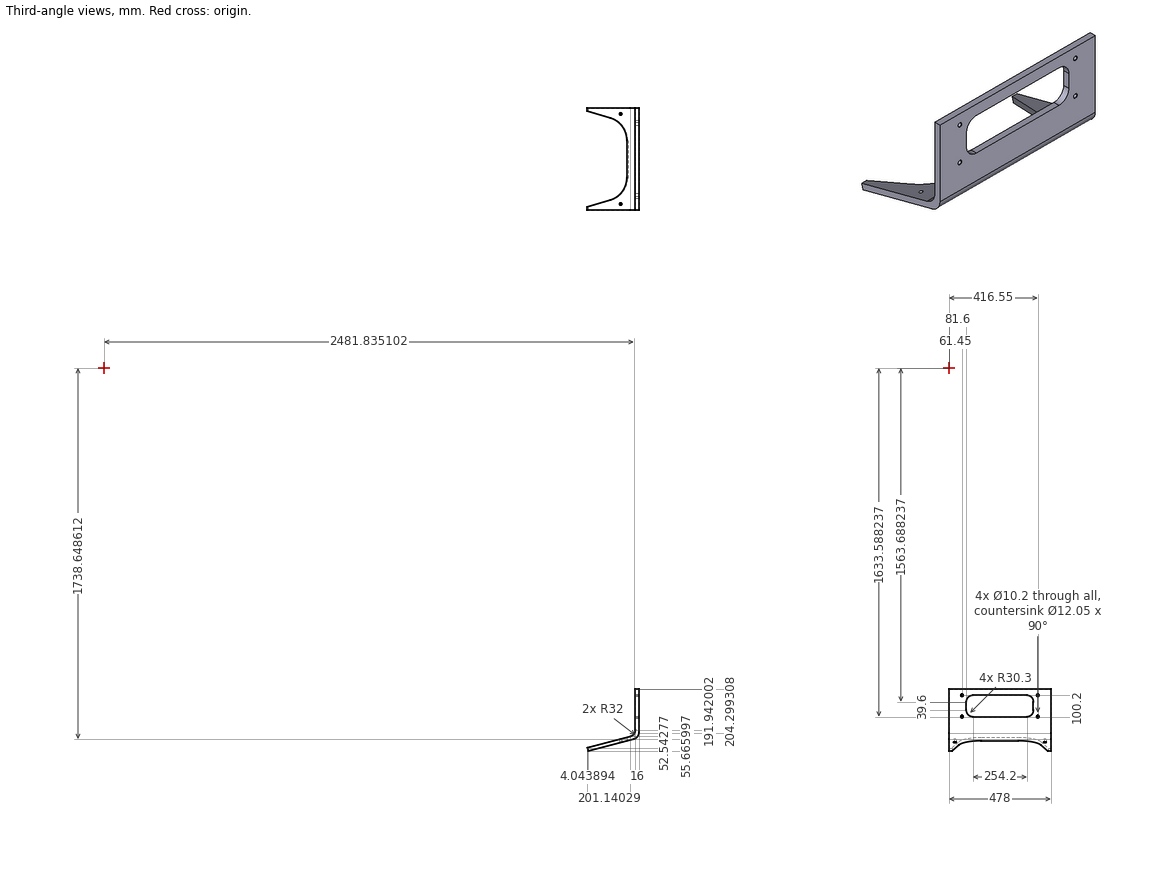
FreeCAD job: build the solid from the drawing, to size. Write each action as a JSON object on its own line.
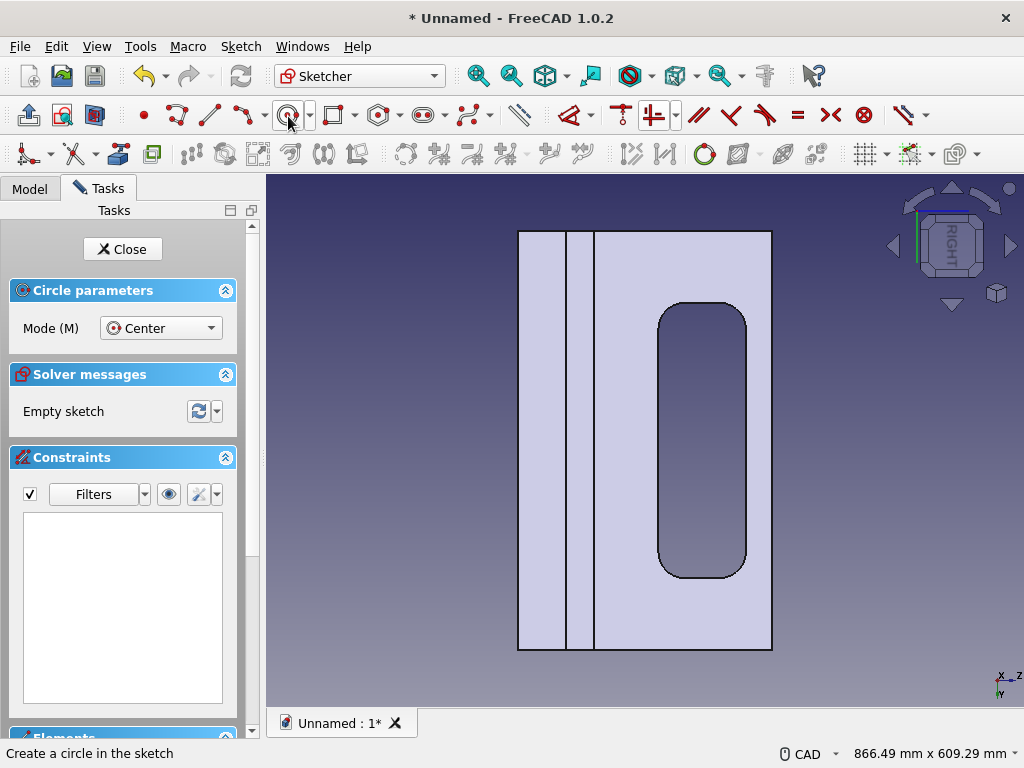
{"action": "scroll", "coordinate": [658, 596], "scroll_direction": "up", "scroll_amount": 9}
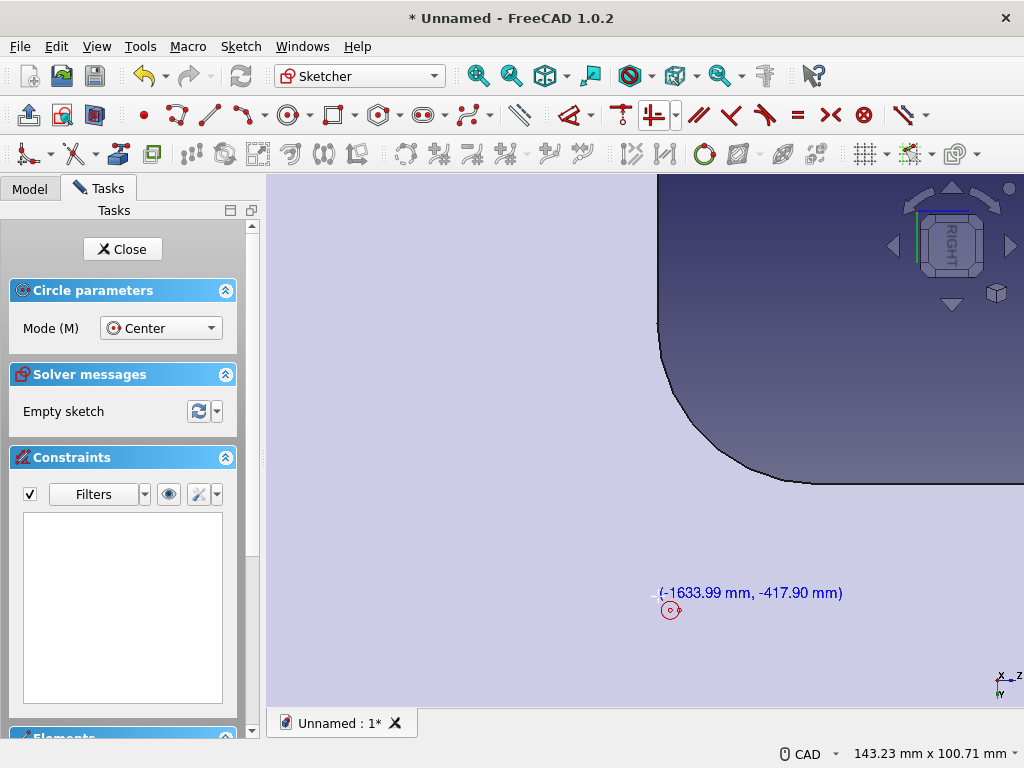
{"action": "scroll", "coordinate": [508, 597], "scroll_direction": "down", "scroll_amount": 9}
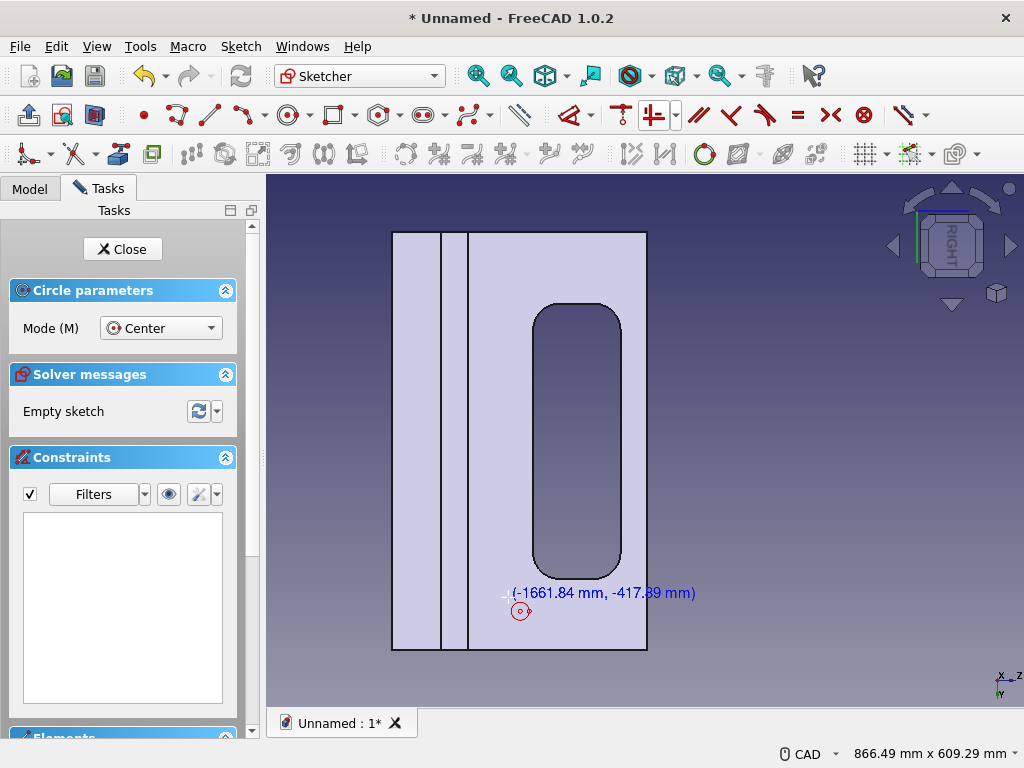
{"action": "left_click", "coordinate": [533, 597]}
{"action": "mouse_move", "coordinate": [536, 594]}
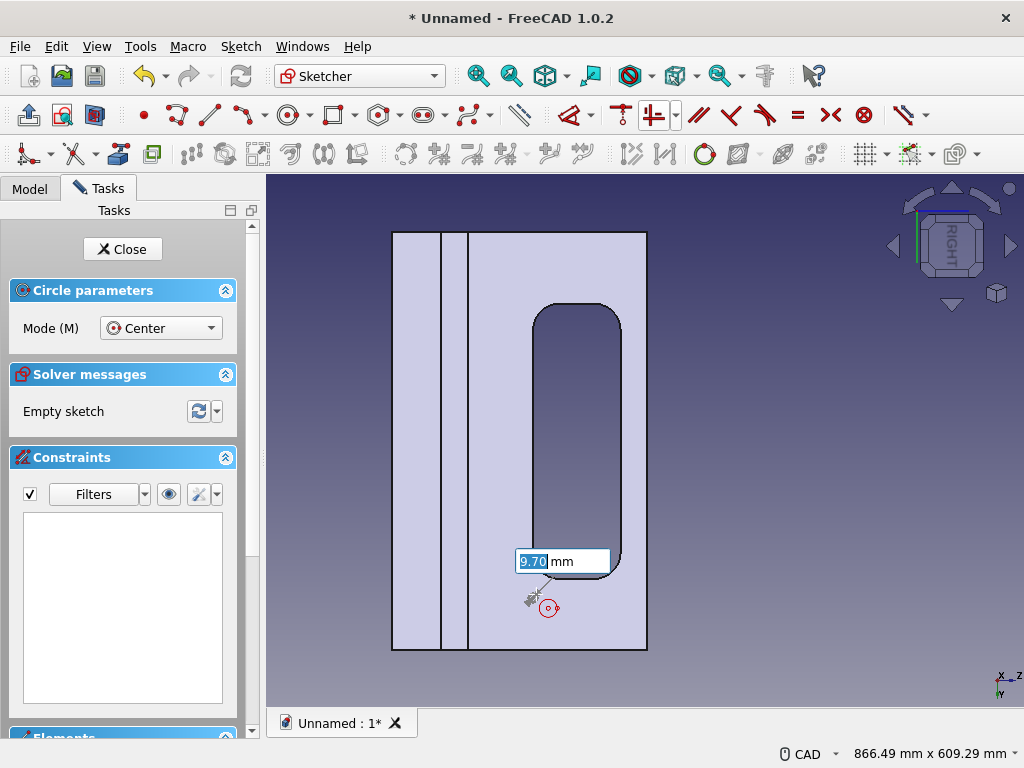
{"action": "type", "text": "10.2"}
{"action": "key", "text": "Return"}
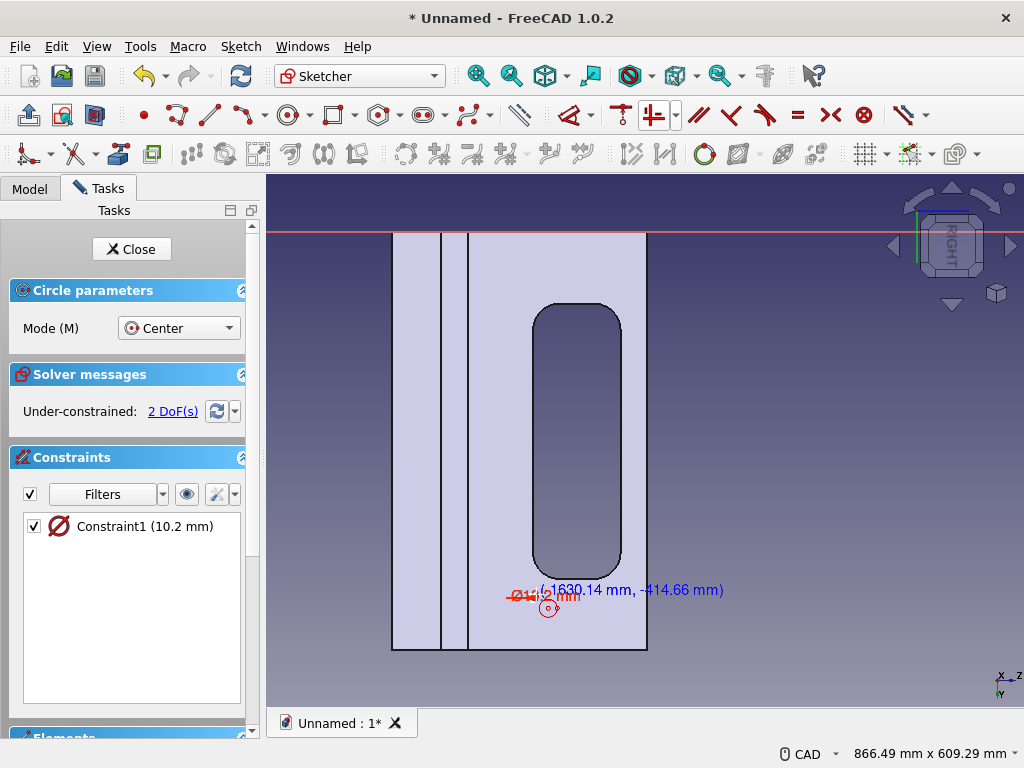
{"action": "scroll", "coordinate": [621, 286], "scroll_direction": "up", "scroll_amount": 9}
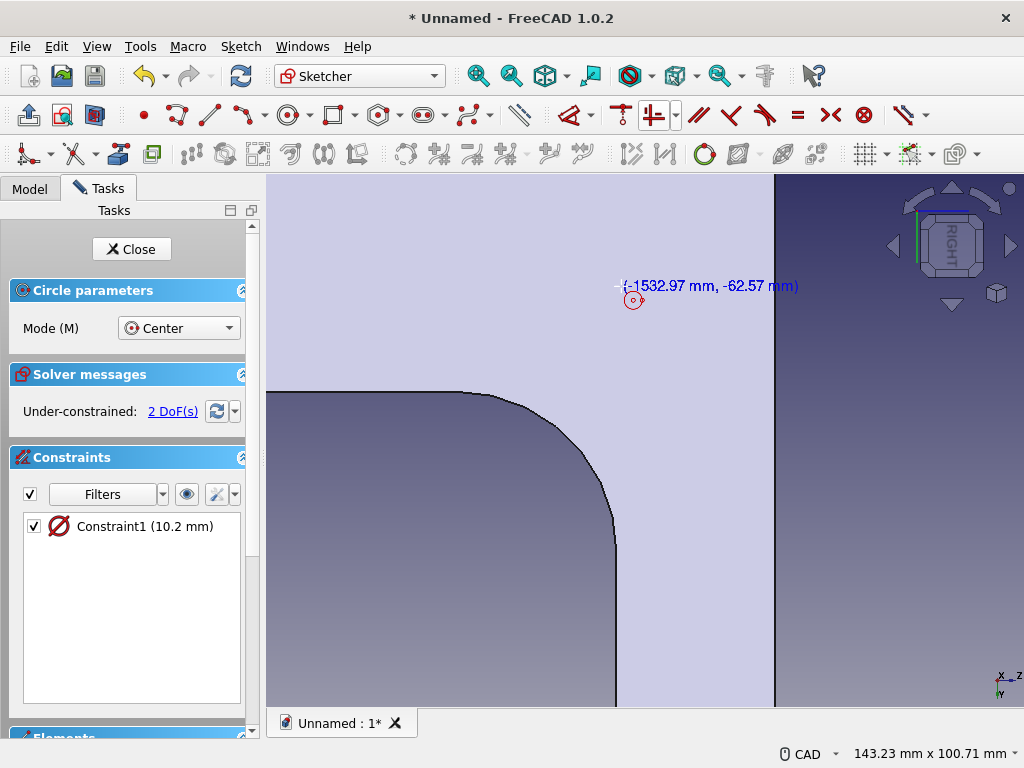
{"action": "scroll", "coordinate": [621, 285], "scroll_direction": "down", "scroll_amount": 9}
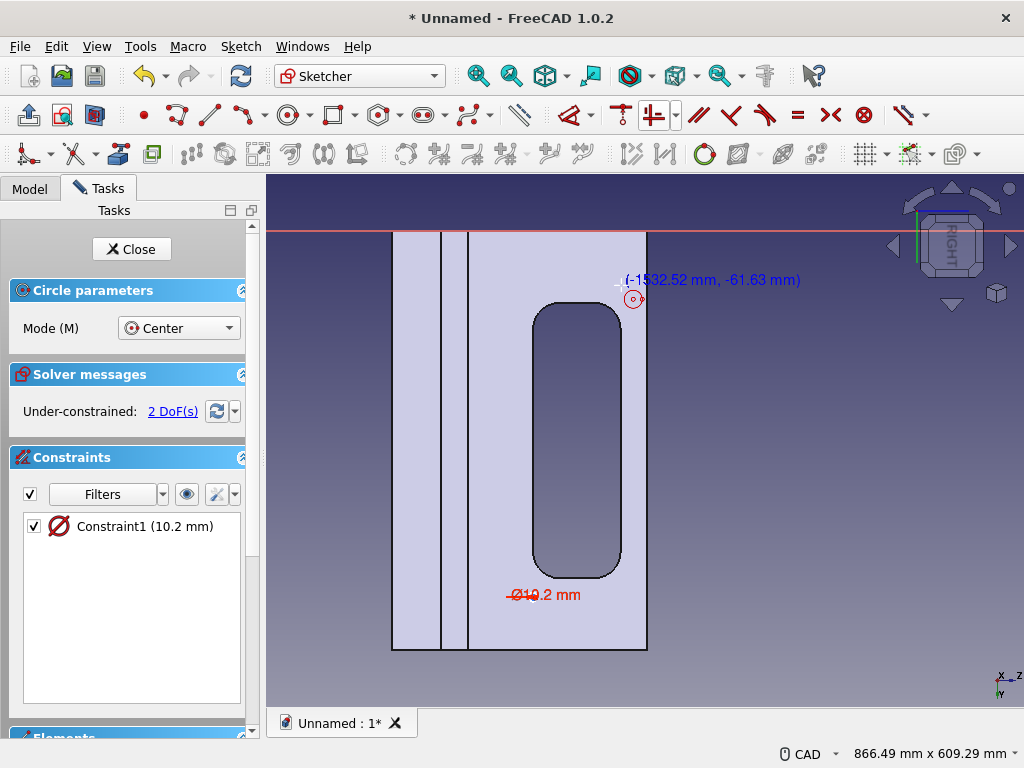
{"action": "left_click", "coordinate": [621, 285]}
{"action": "mouse_move", "coordinate": [624, 282]}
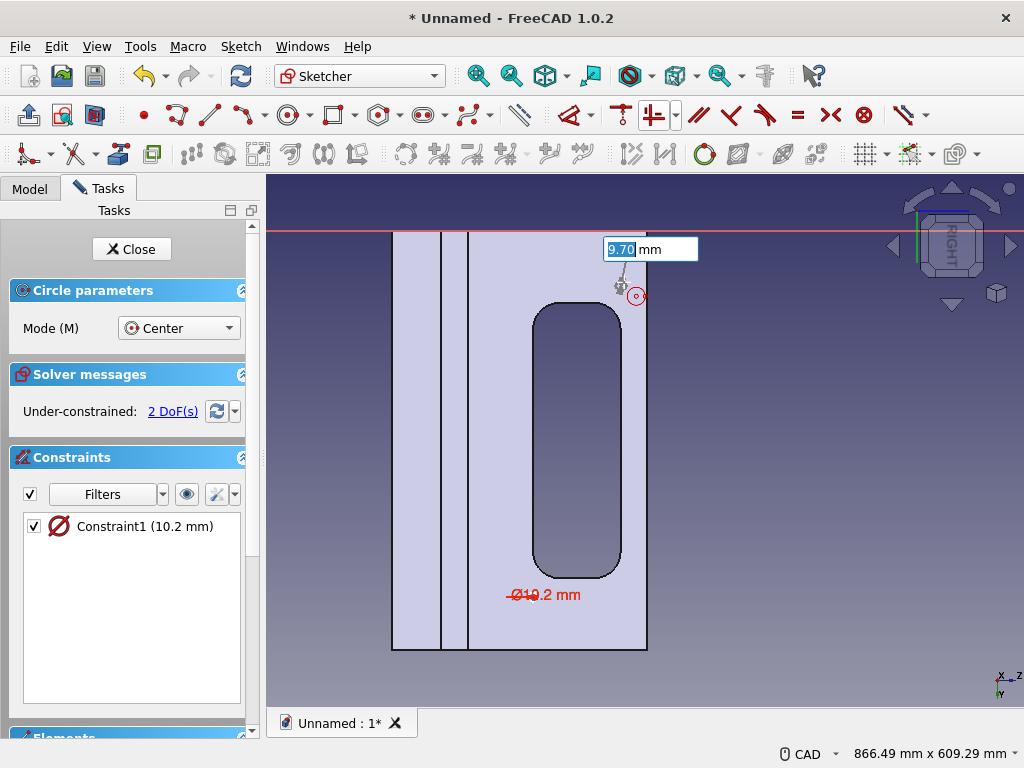
{"action": "type", "text": "10.2"}
{"action": "key", "text": "Return"}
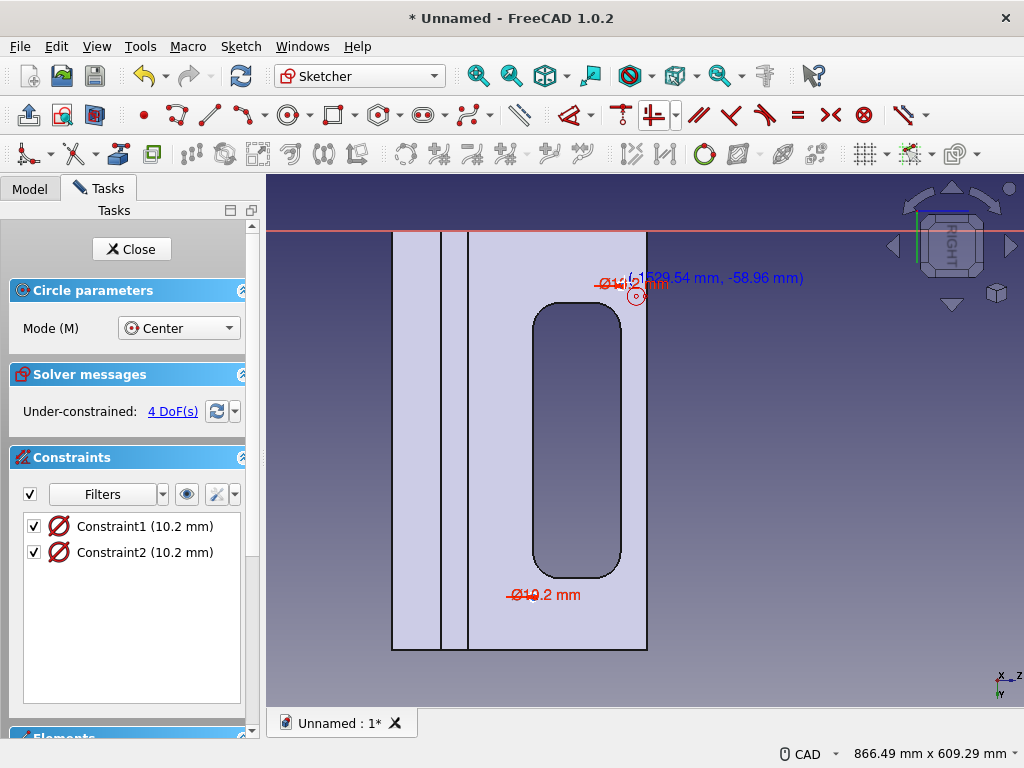
{"action": "scroll", "coordinate": [621, 596], "scroll_direction": "up", "scroll_amount": 9}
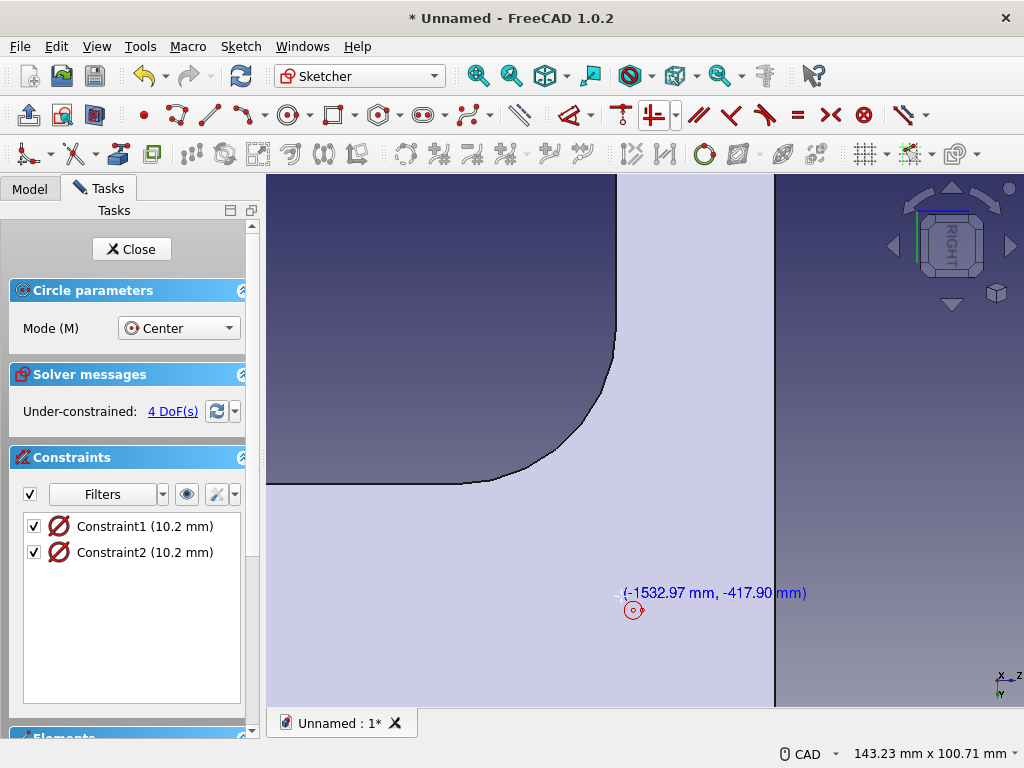
{"action": "scroll", "coordinate": [621, 597], "scroll_direction": "down", "scroll_amount": 9}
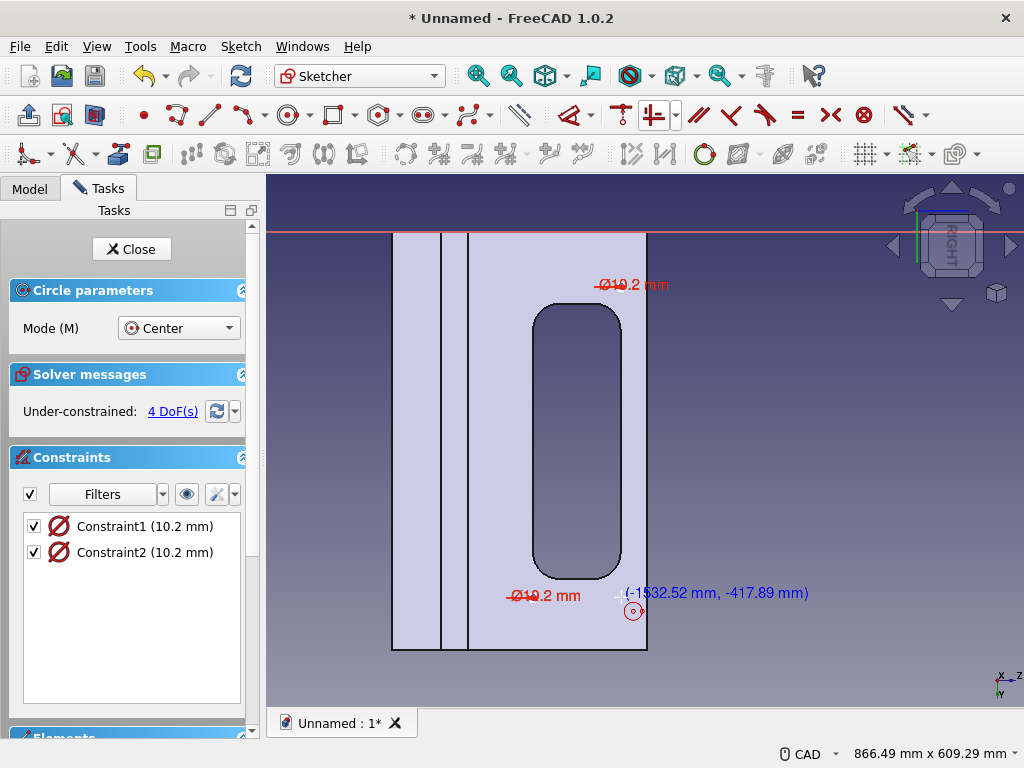
{"action": "left_click", "coordinate": [621, 597]}
{"action": "mouse_move", "coordinate": [624, 594]}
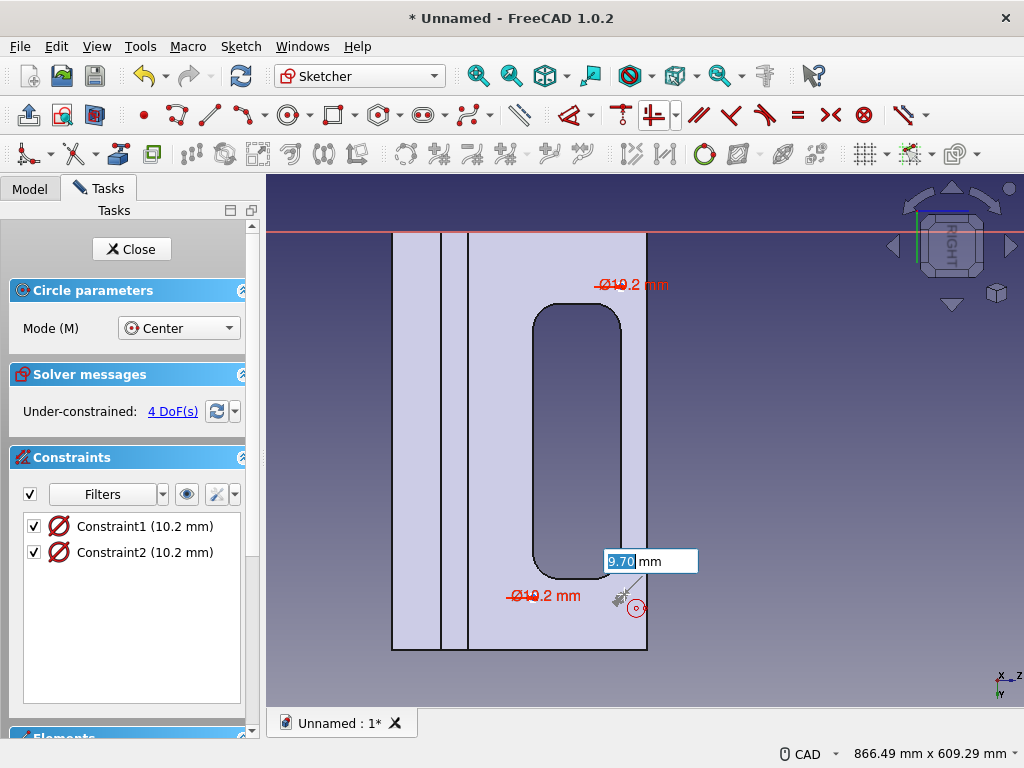
{"action": "type", "text": "10.2"}
{"action": "key", "text": "Return"}